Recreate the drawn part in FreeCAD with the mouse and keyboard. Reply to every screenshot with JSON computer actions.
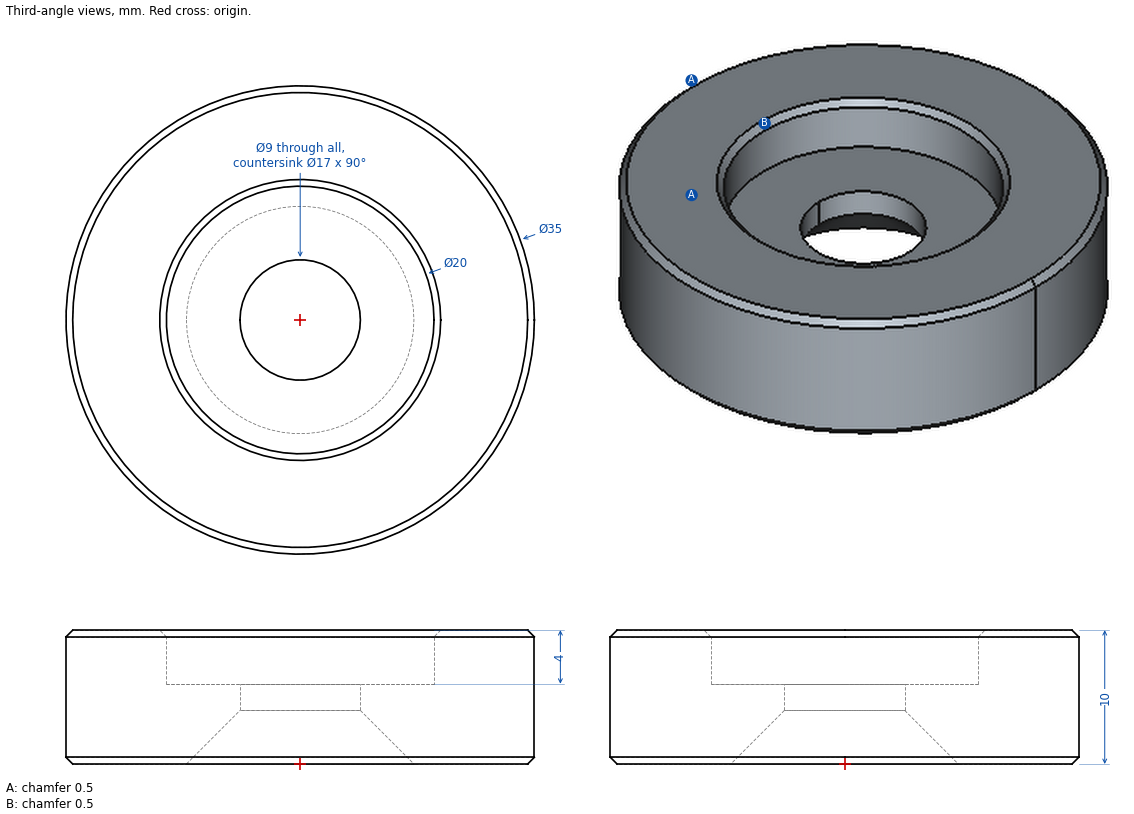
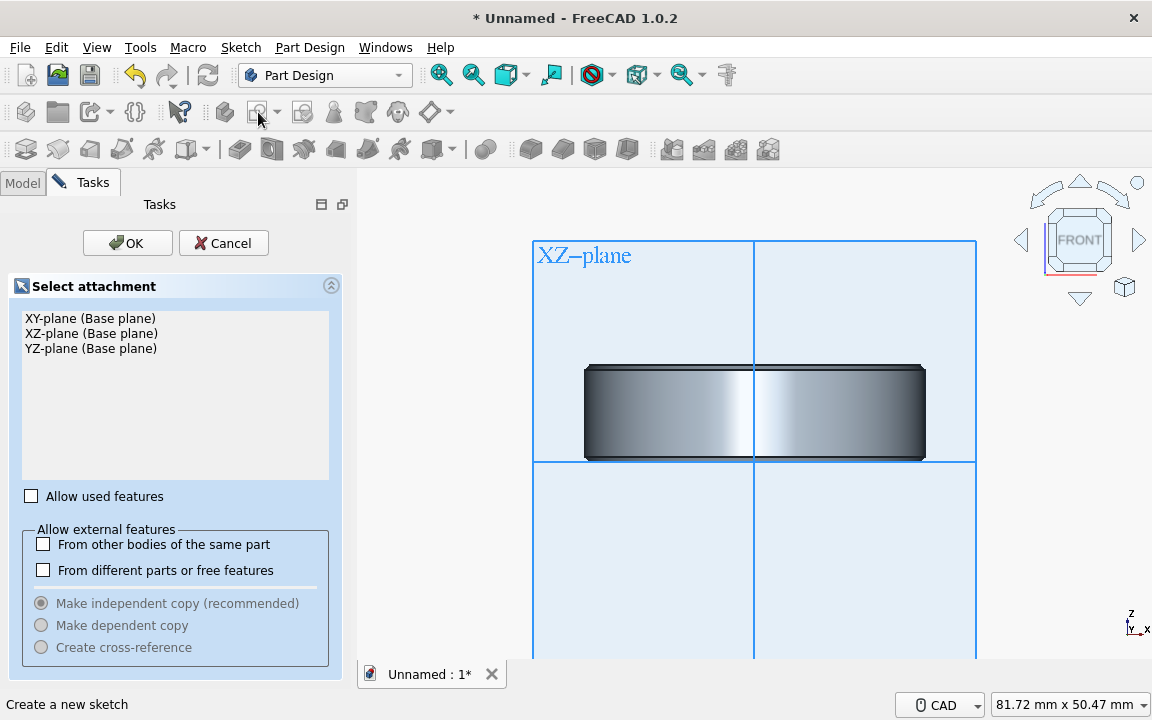
{"action": "left_click", "coordinate": [82, 318]}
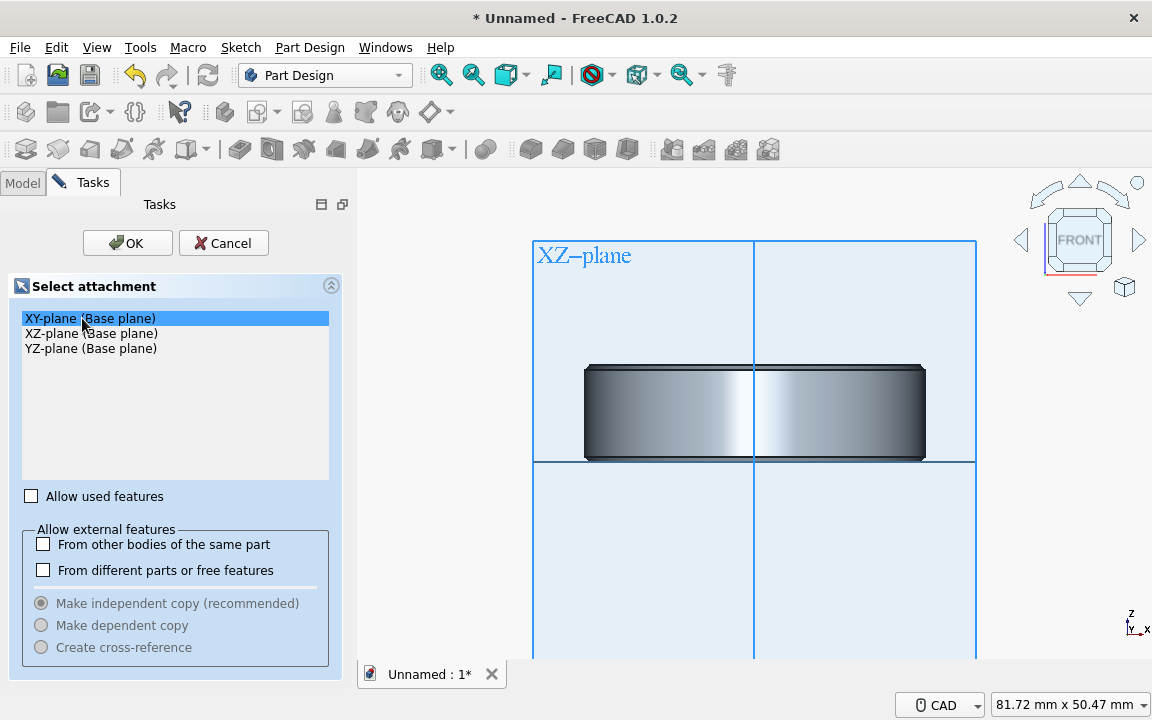
{"action": "left_click", "coordinate": [128, 243]}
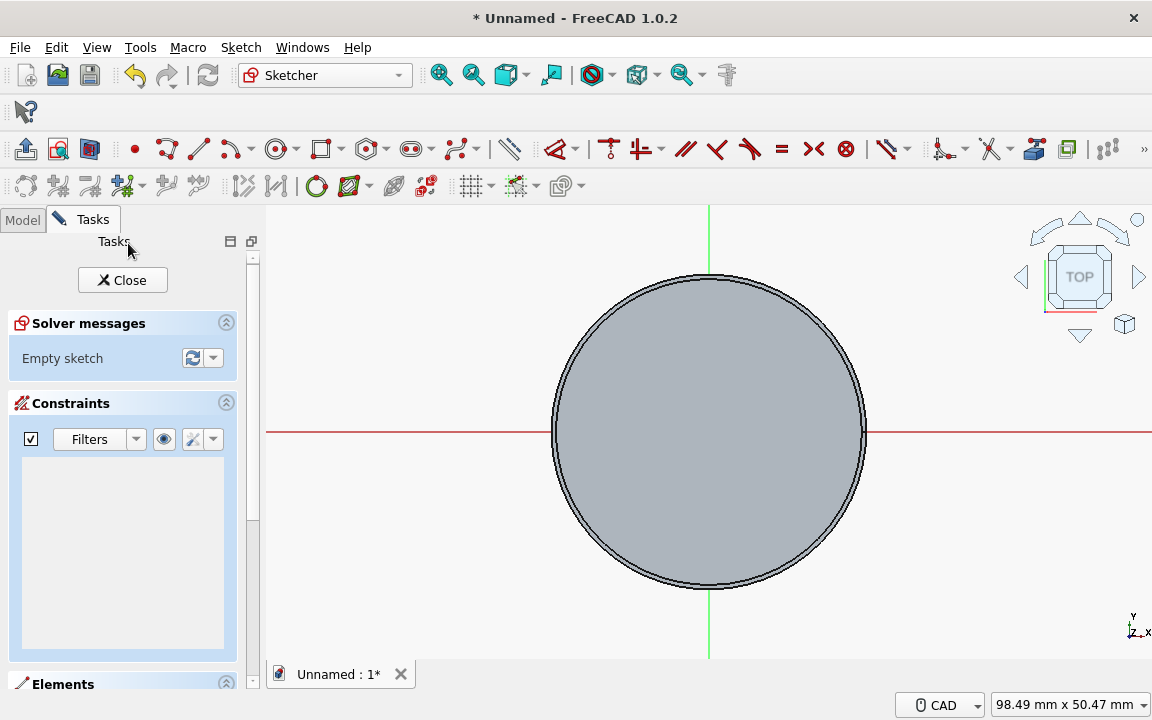
{"action": "left_click", "coordinate": [90, 150]}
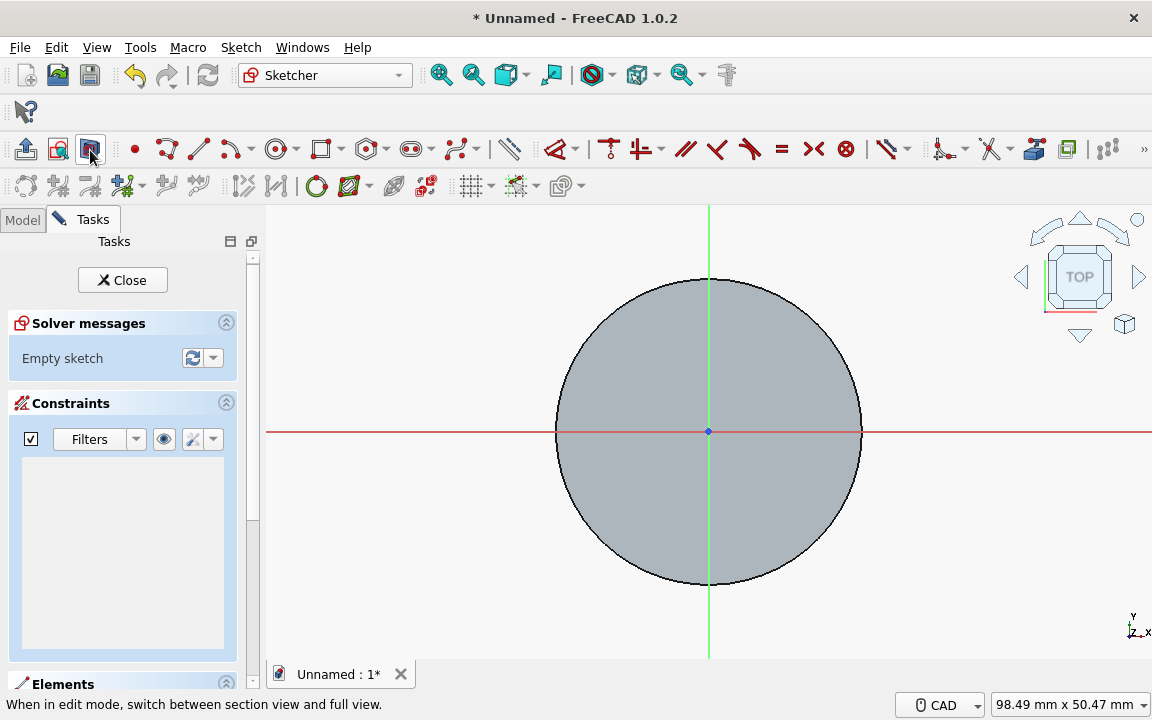
{"action": "scroll", "coordinate": [738, 432], "scroll_direction": "up", "scroll_amount": 6}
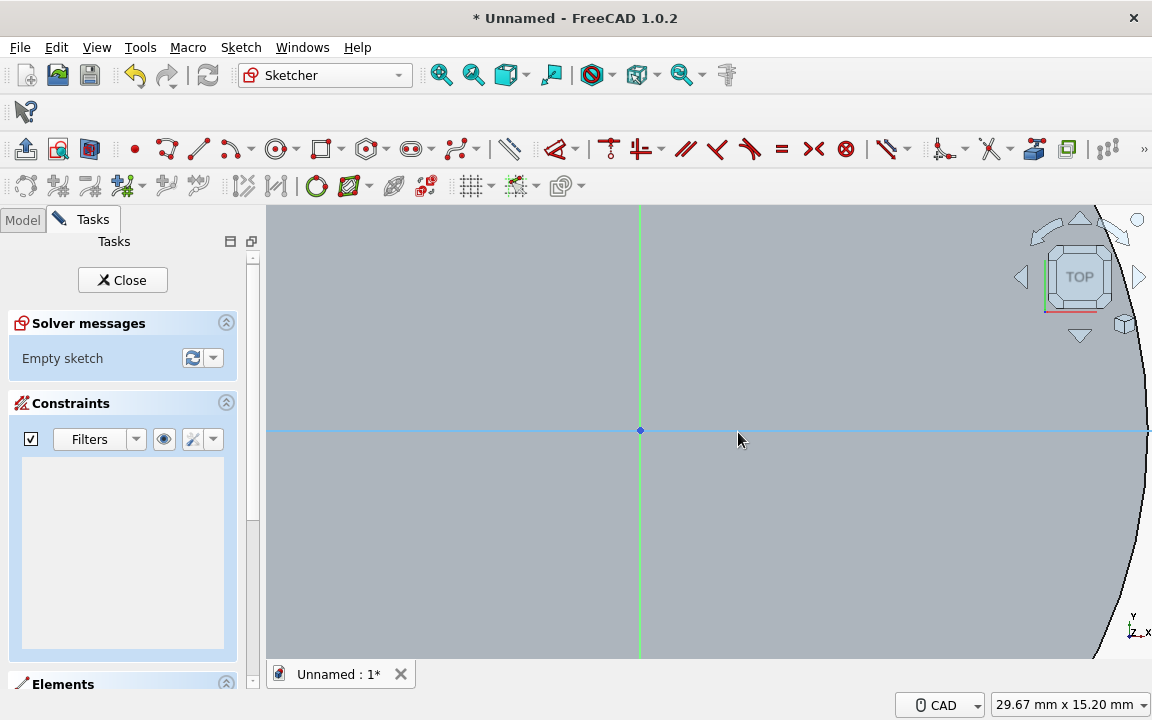
{"action": "left_click", "coordinate": [276, 150]}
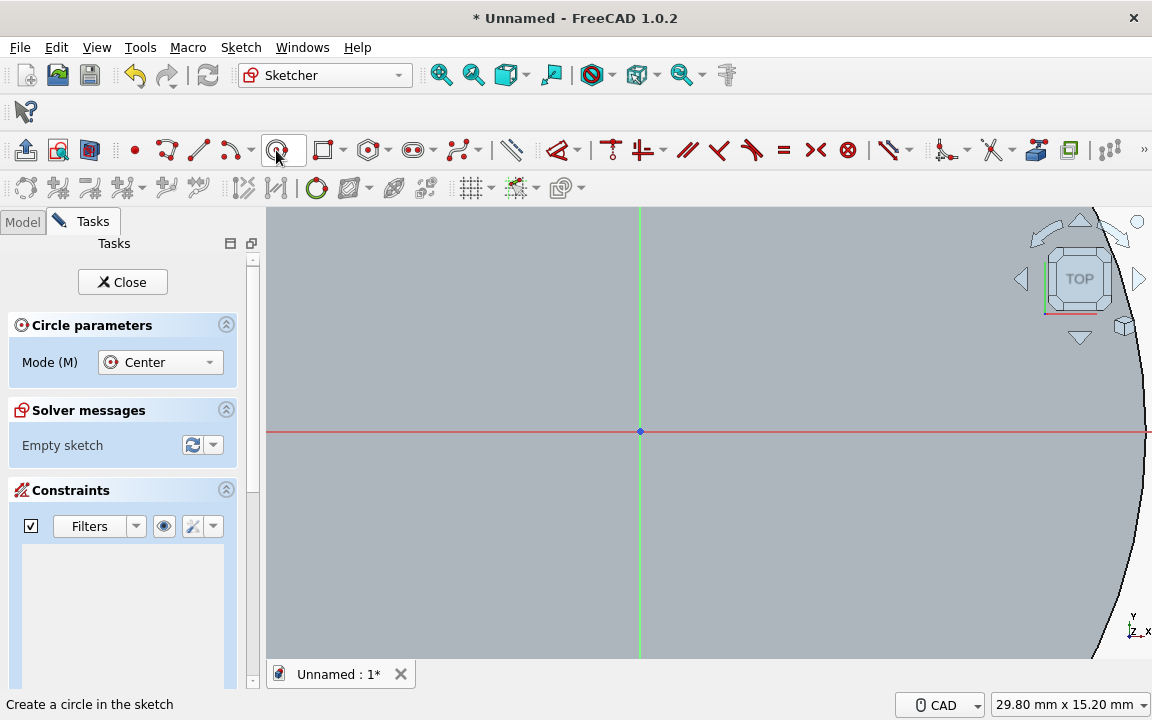
{"action": "left_click", "coordinate": [640, 432]}
{"action": "mouse_move", "coordinate": [735, 337]}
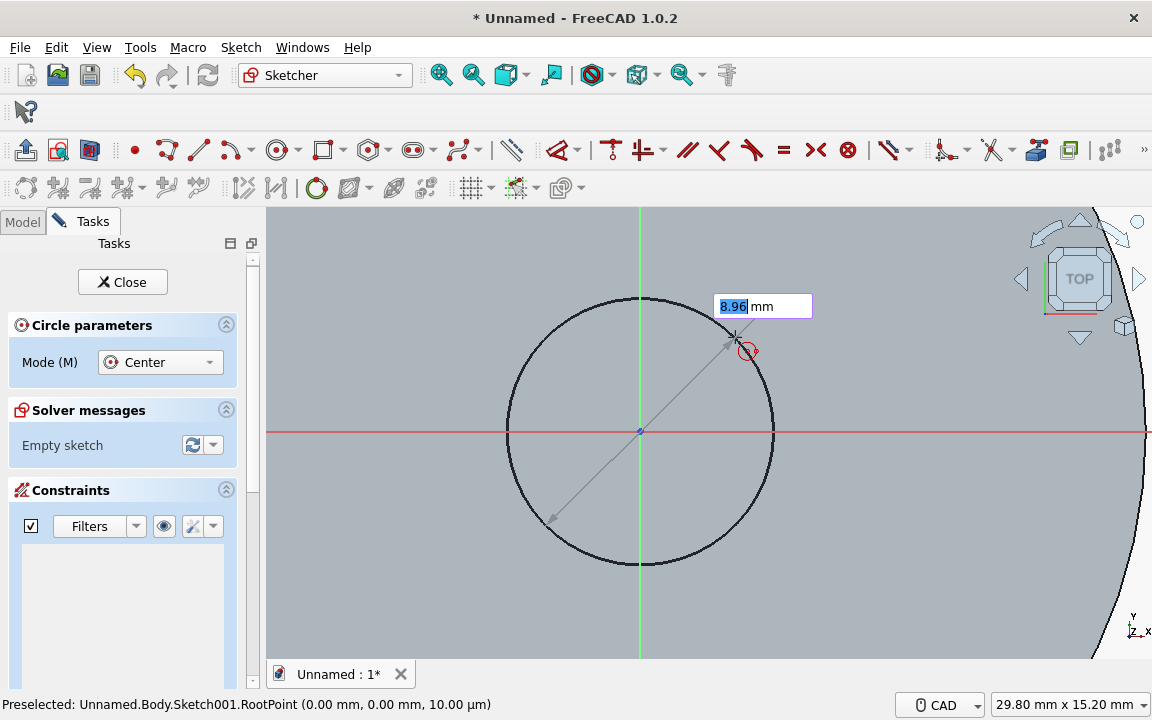
{"action": "type", "text": "9"}
{"action": "key", "text": "Return"}
{"action": "key", "text": "Escape"}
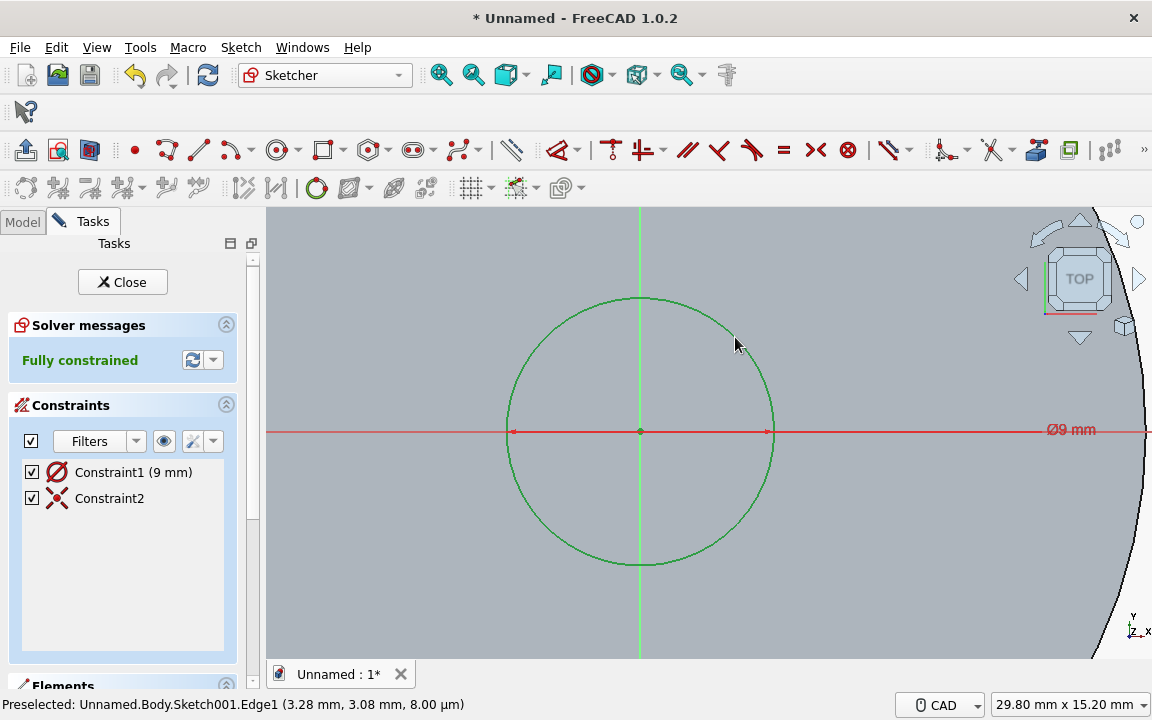
{"action": "left_click", "coordinate": [123, 282]}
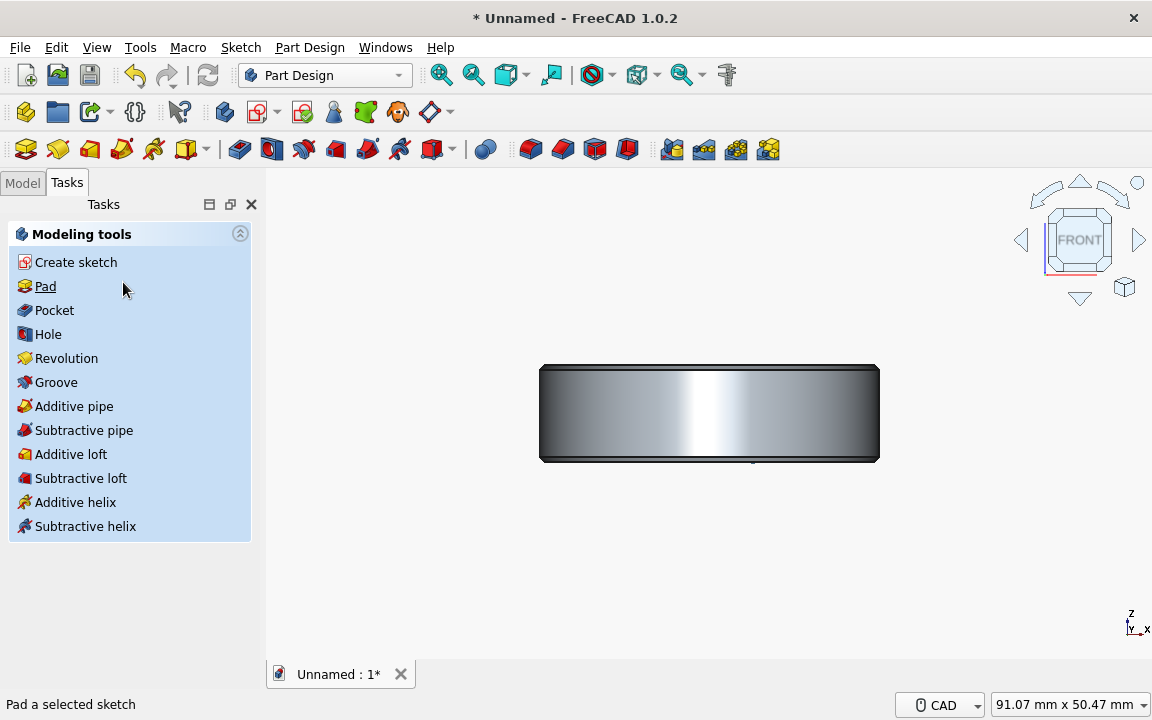
{"action": "left_click", "coordinate": [272, 150]}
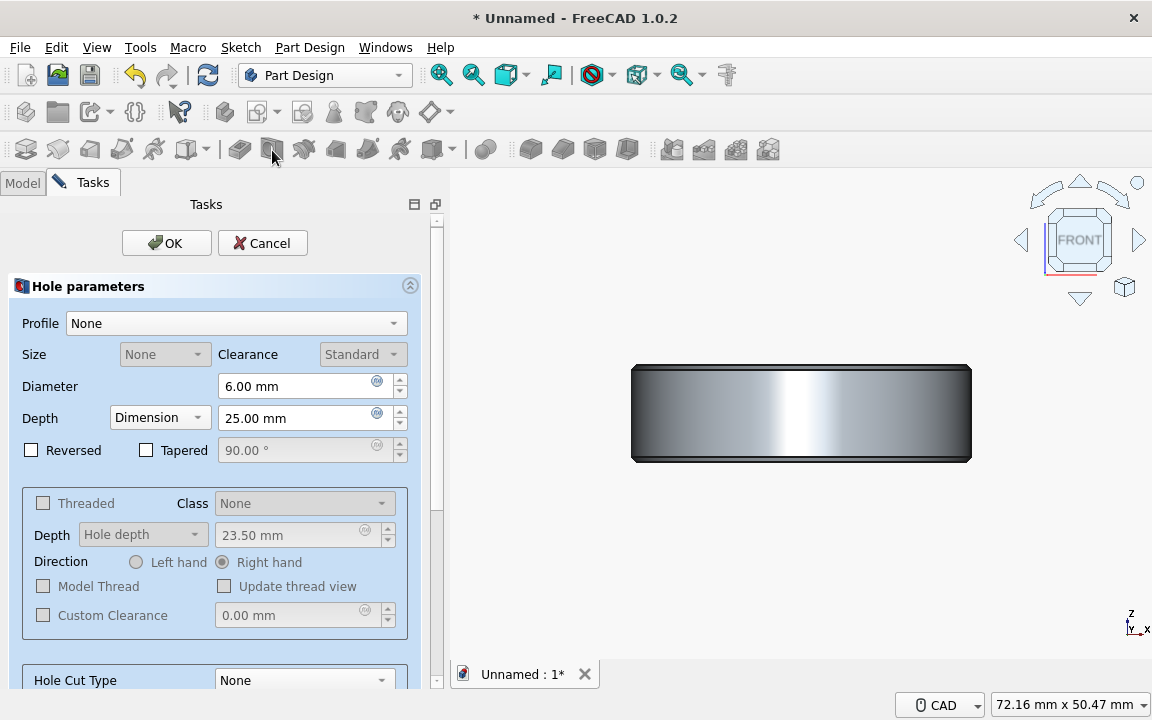
{"action": "triple_click", "coordinate": [305, 386]}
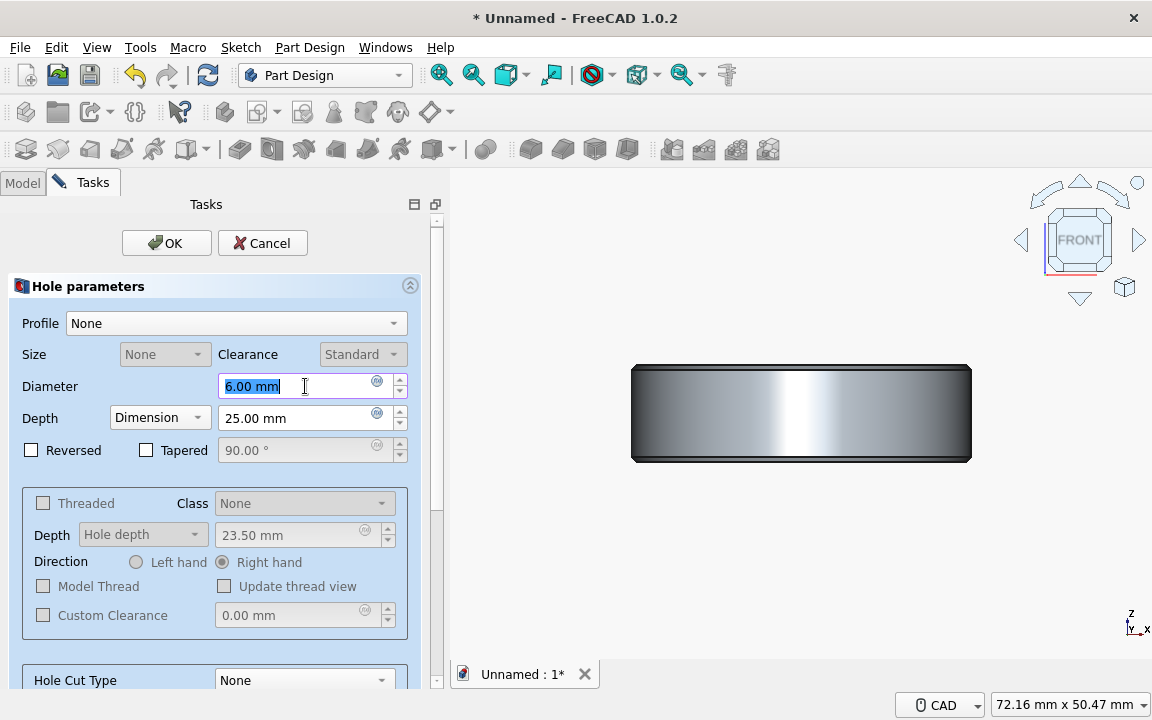
{"action": "type", "text": "9"}
{"action": "key", "text": "Tab"}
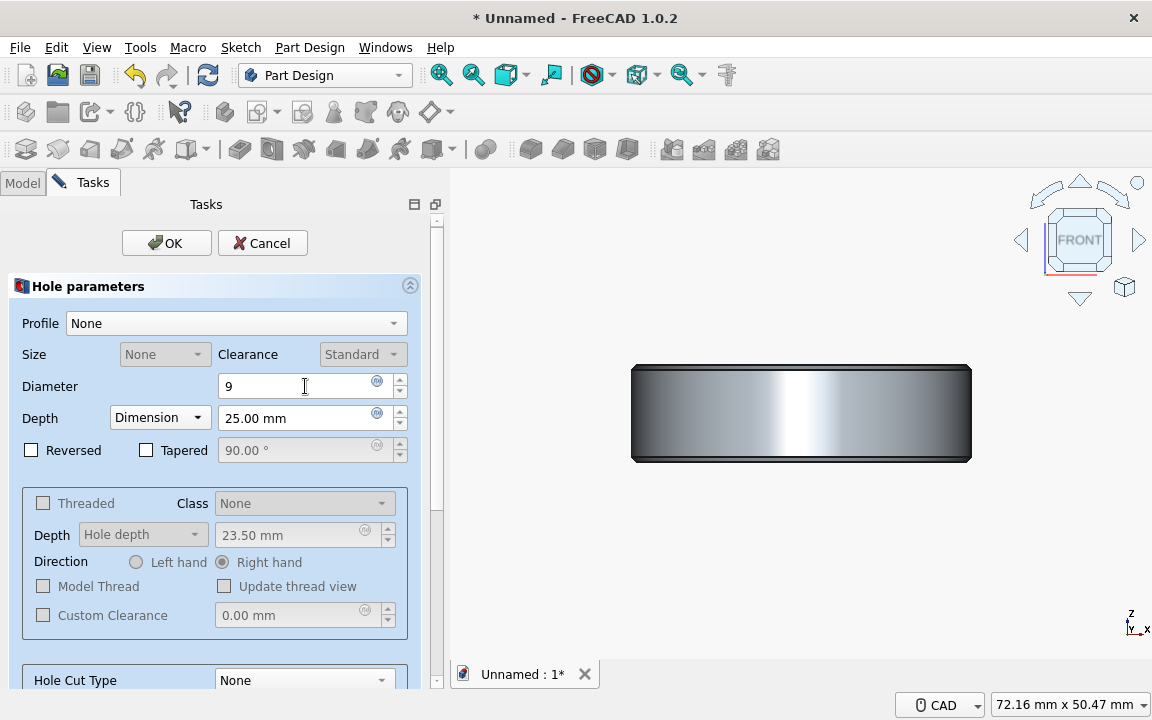
{"action": "left_click", "coordinate": [161, 418]}